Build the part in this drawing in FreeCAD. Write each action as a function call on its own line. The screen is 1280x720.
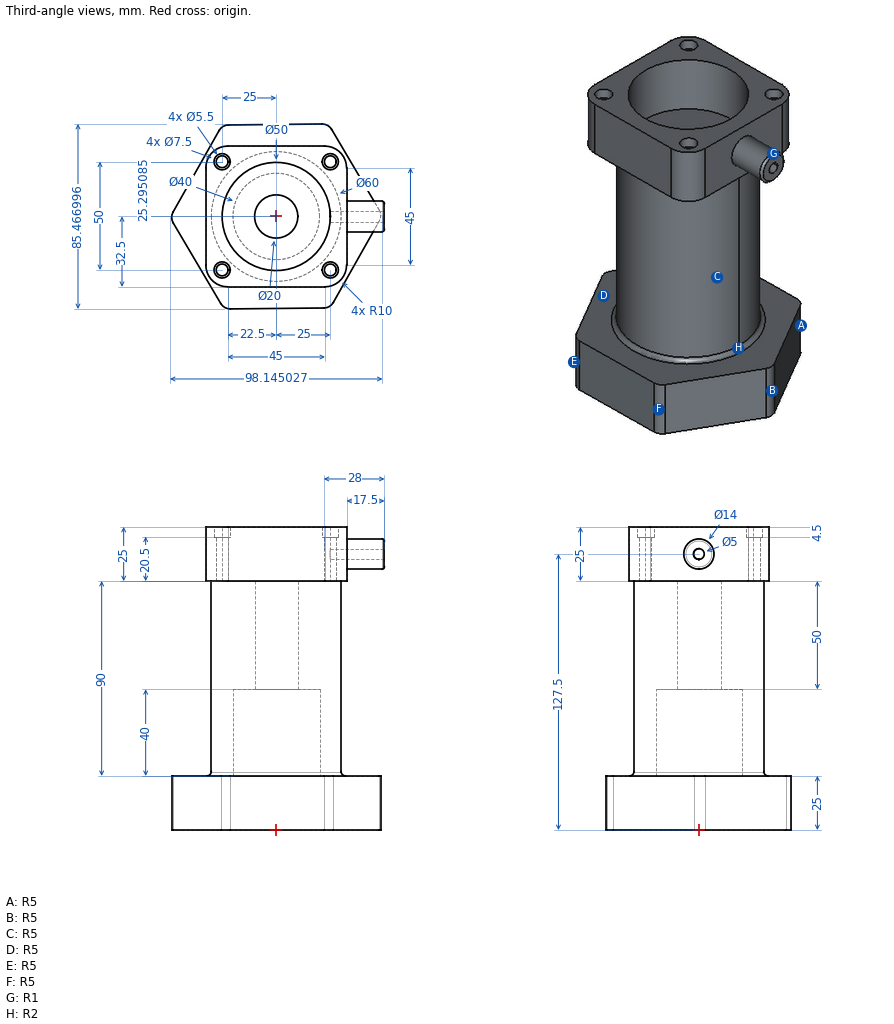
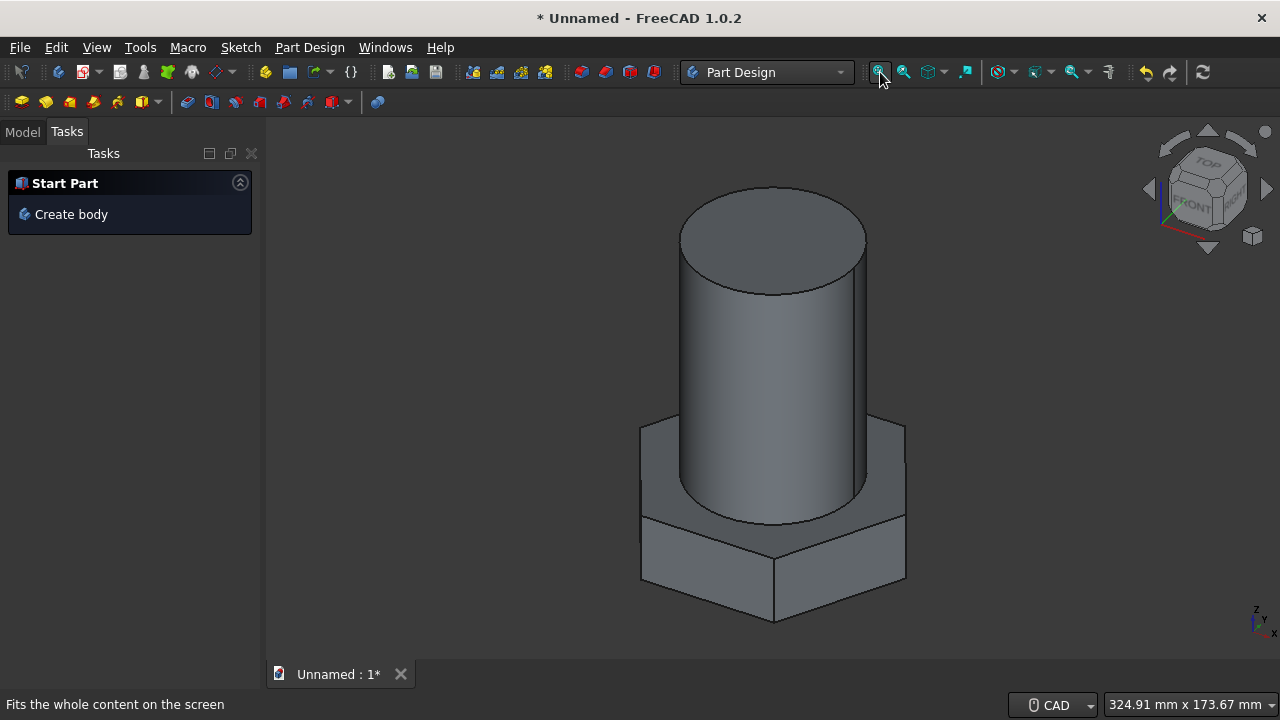
click(773, 240)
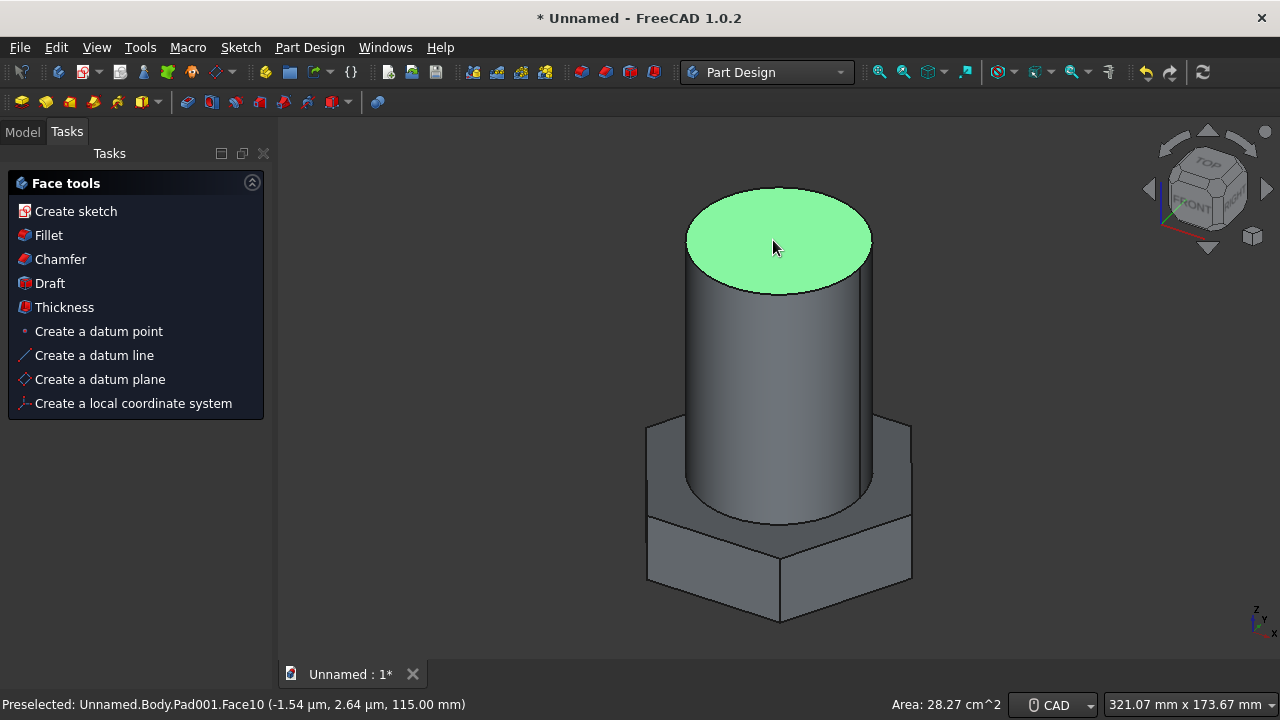
click(84, 72)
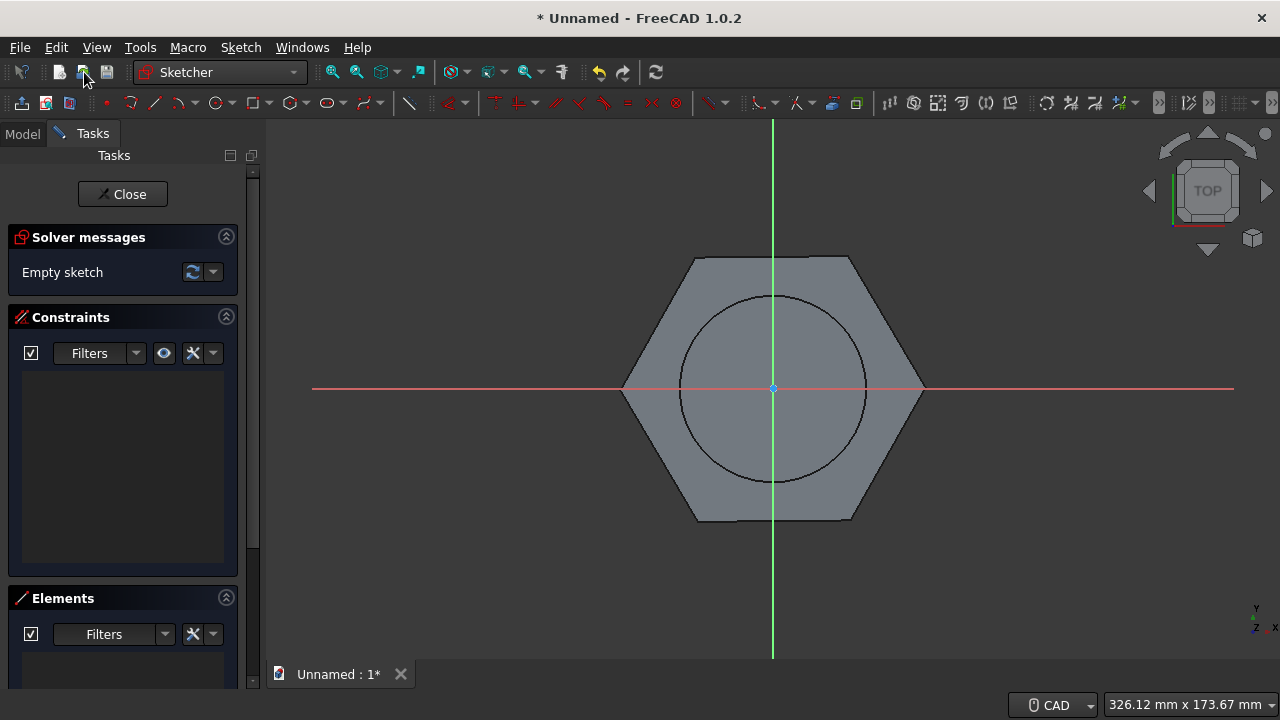
scroll(856, 389, up, 3)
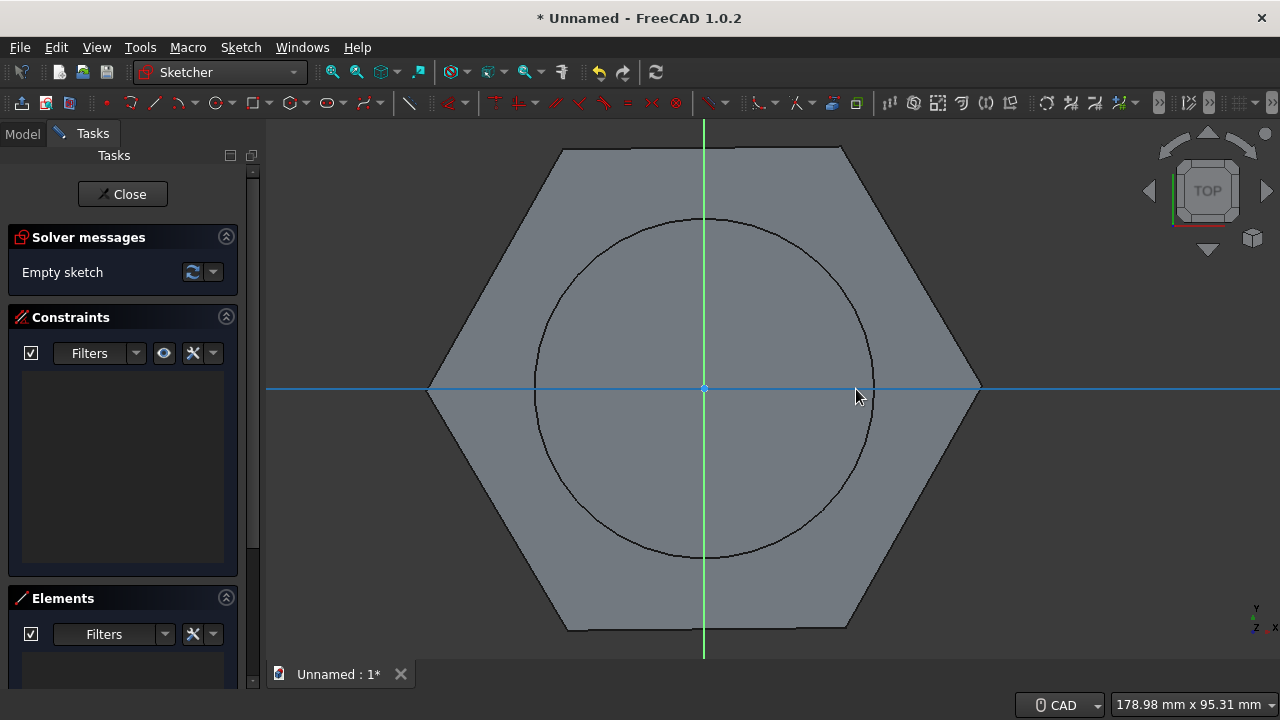
click(156, 104)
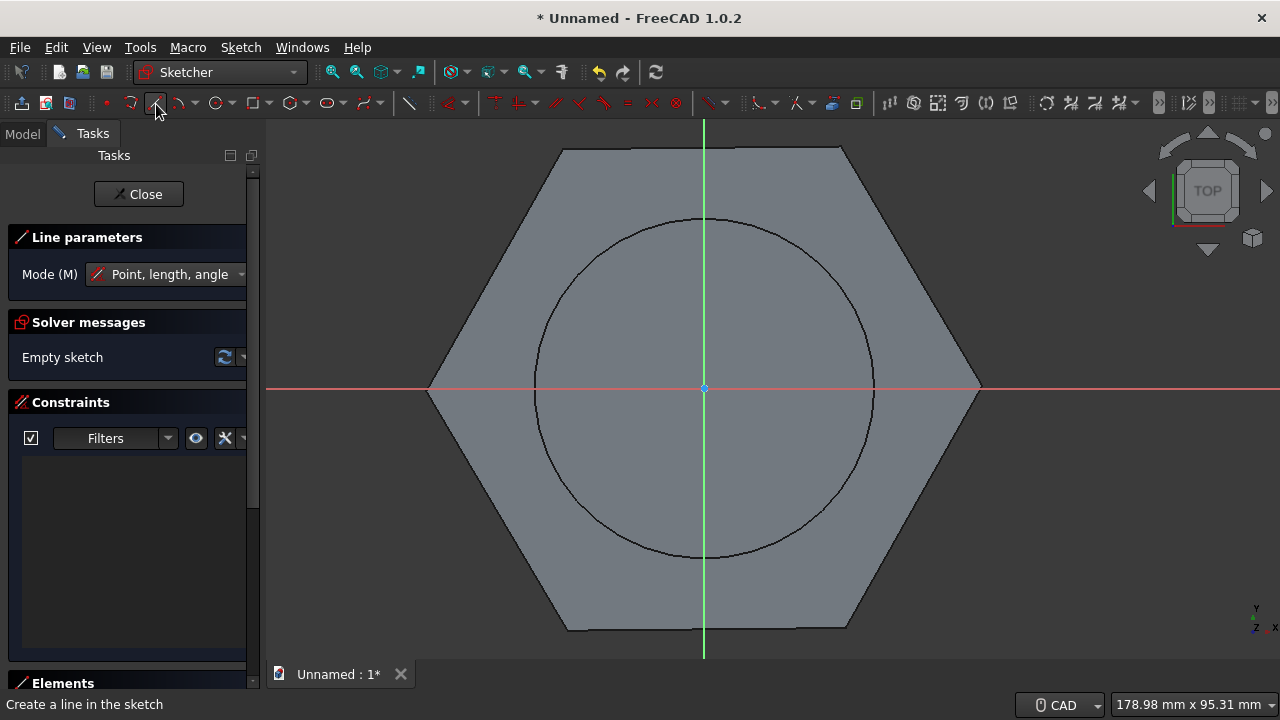
click(577, 573)
click(832, 573)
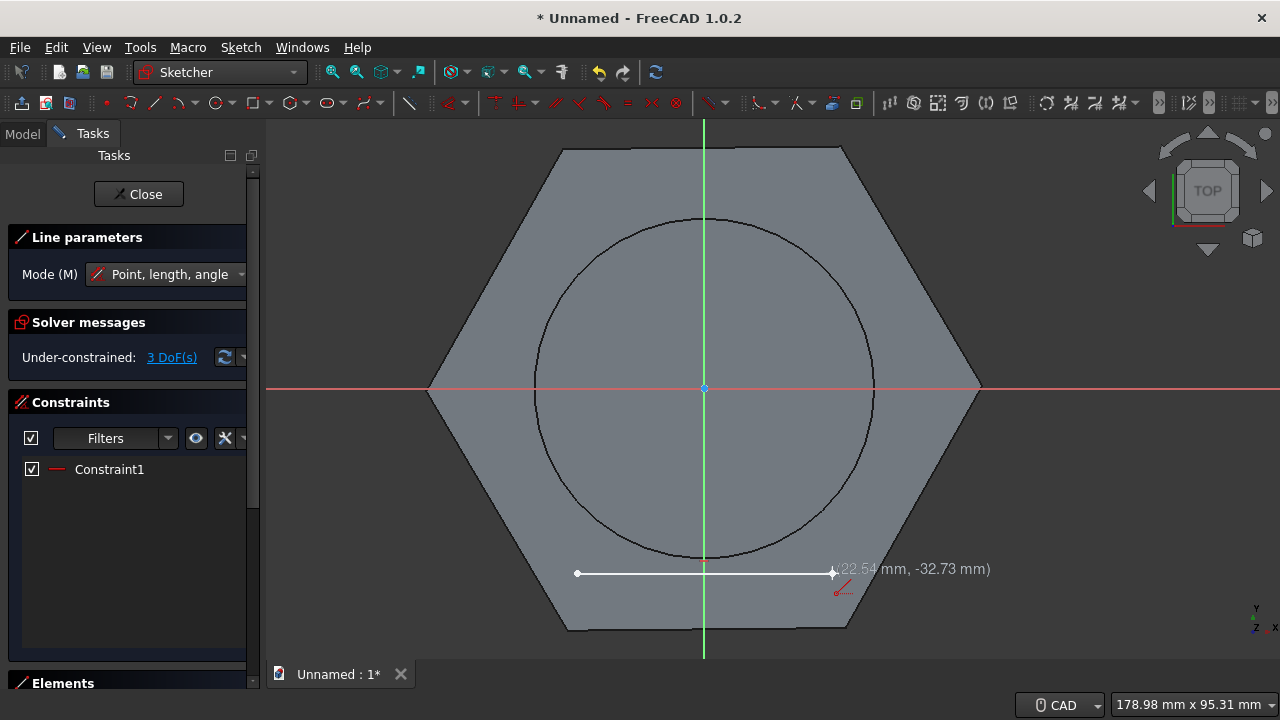
click(888, 516)
click(888, 261)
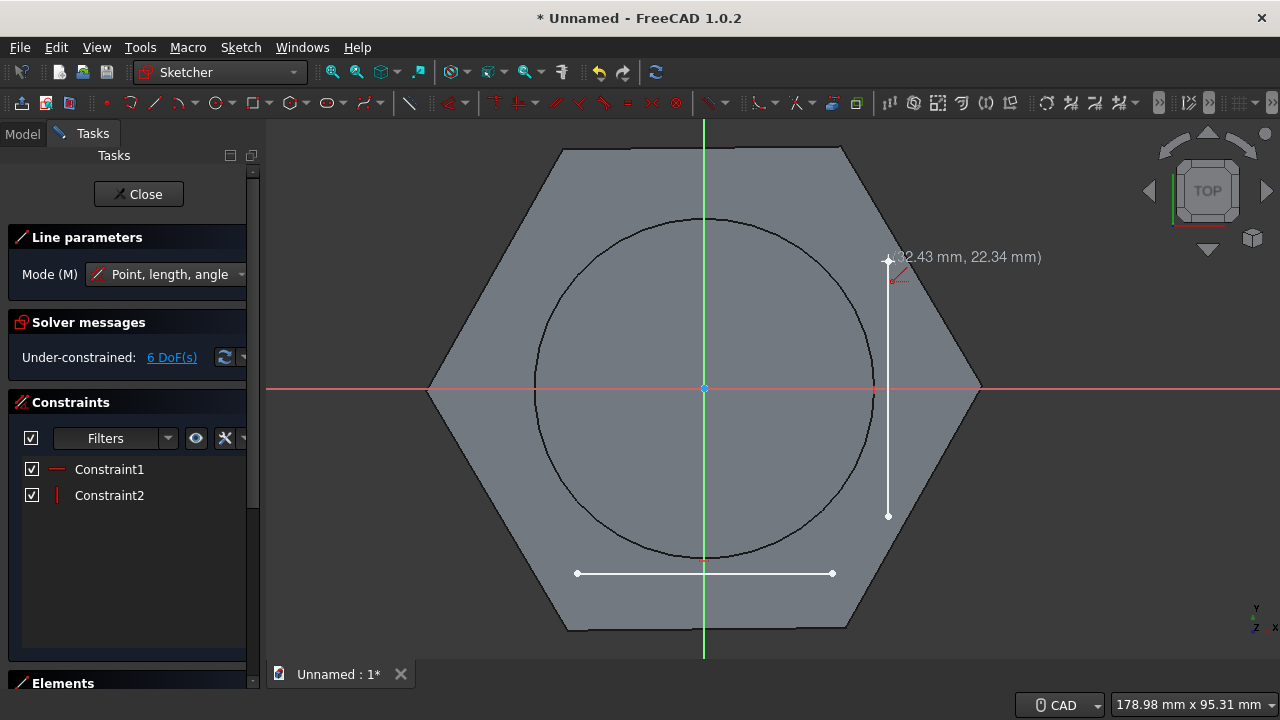
click(832, 204)
click(577, 204)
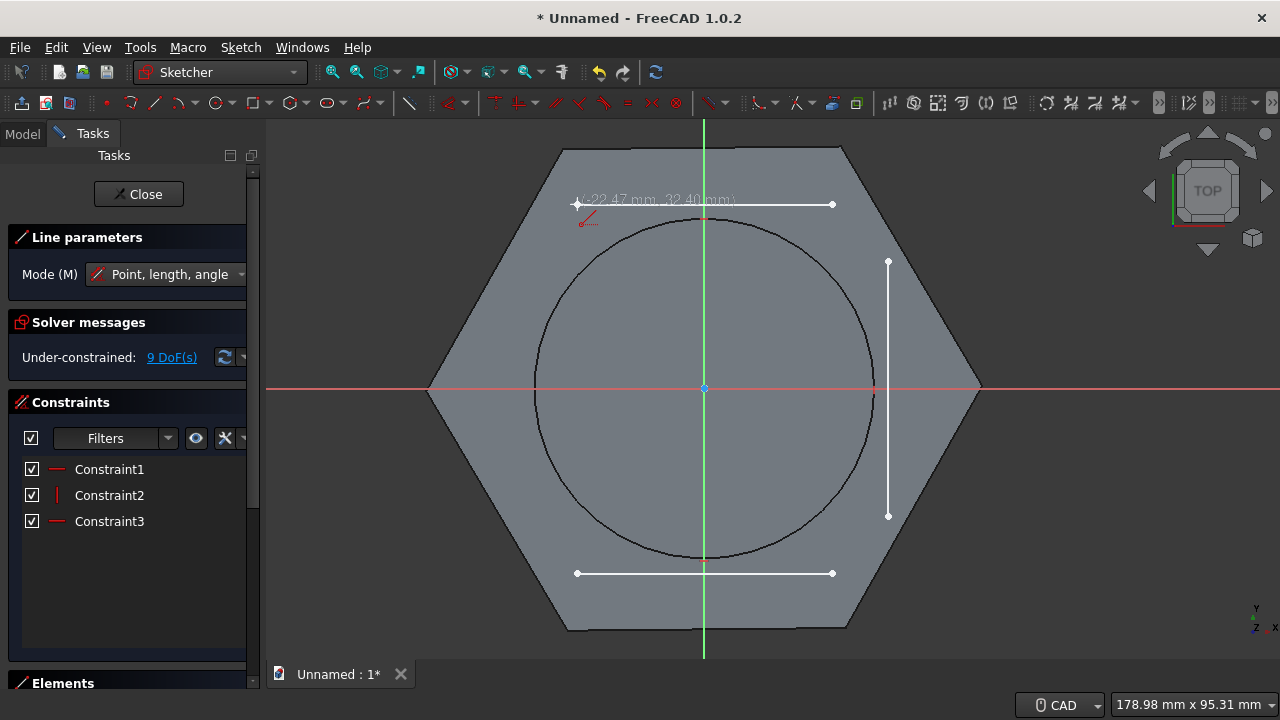
click(520, 261)
click(520, 516)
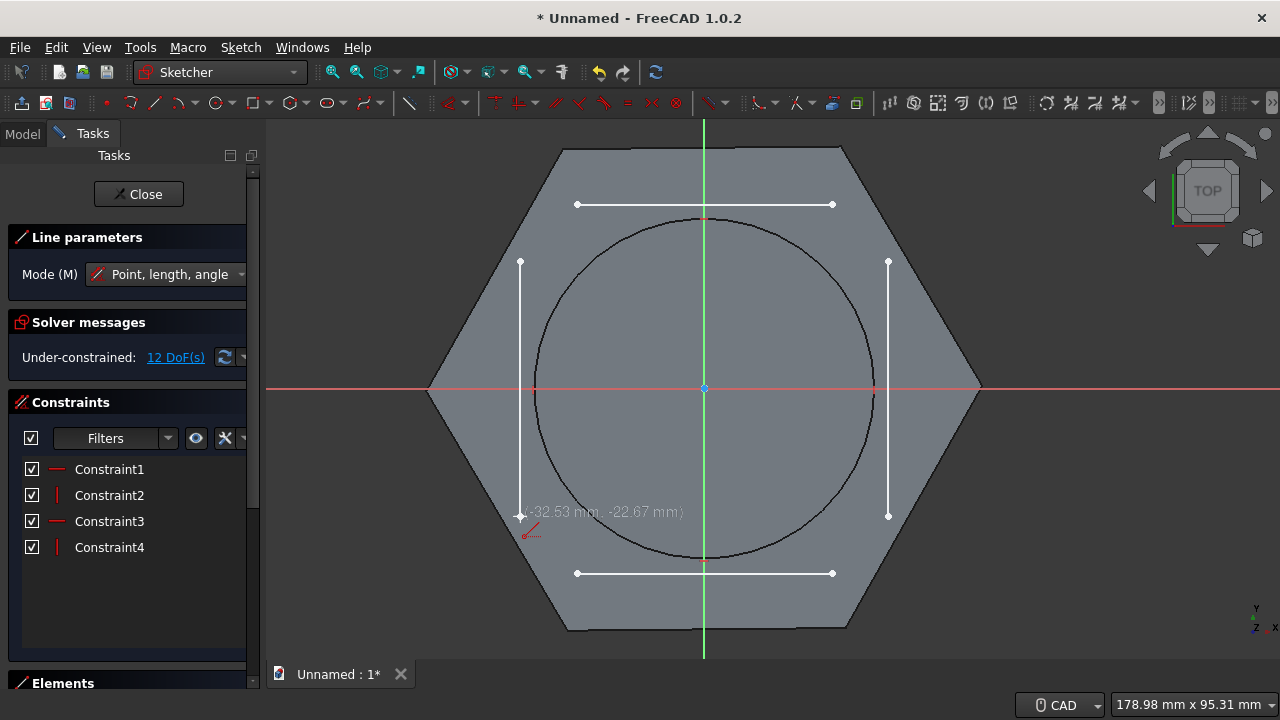
key(g)
key(3)
key(a)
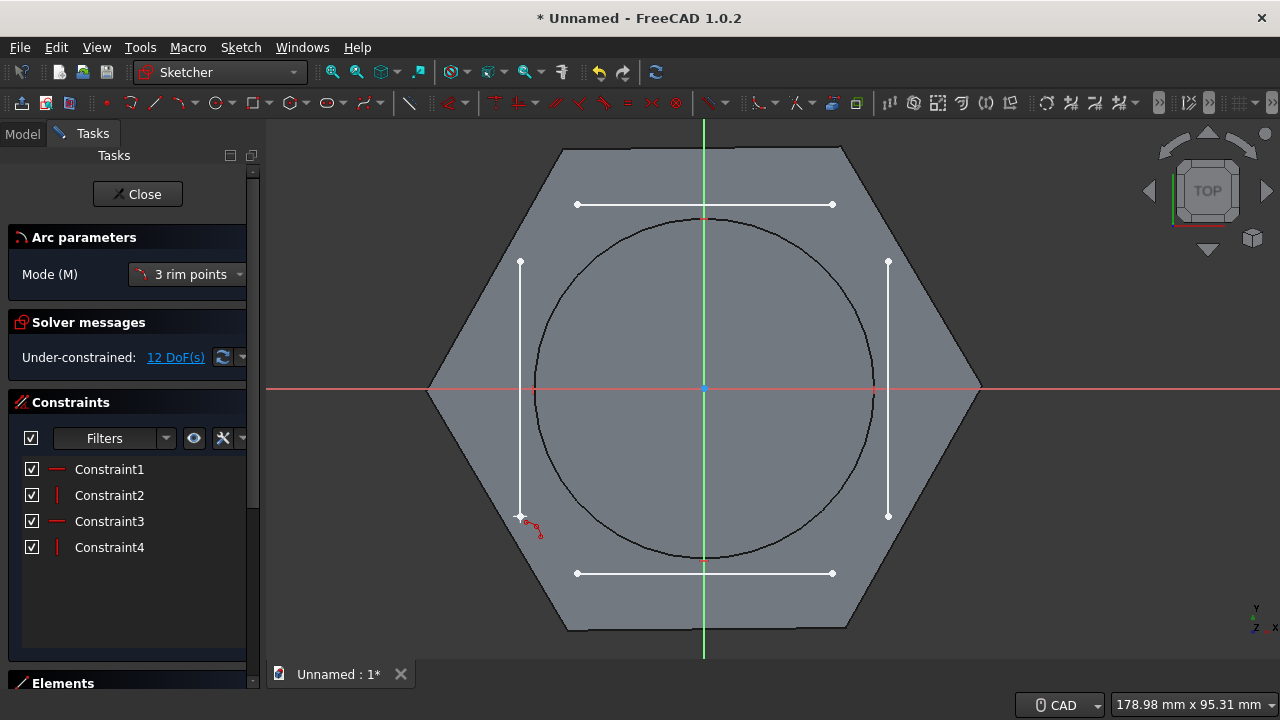
click(832, 574)
click(888, 517)
click(872, 556)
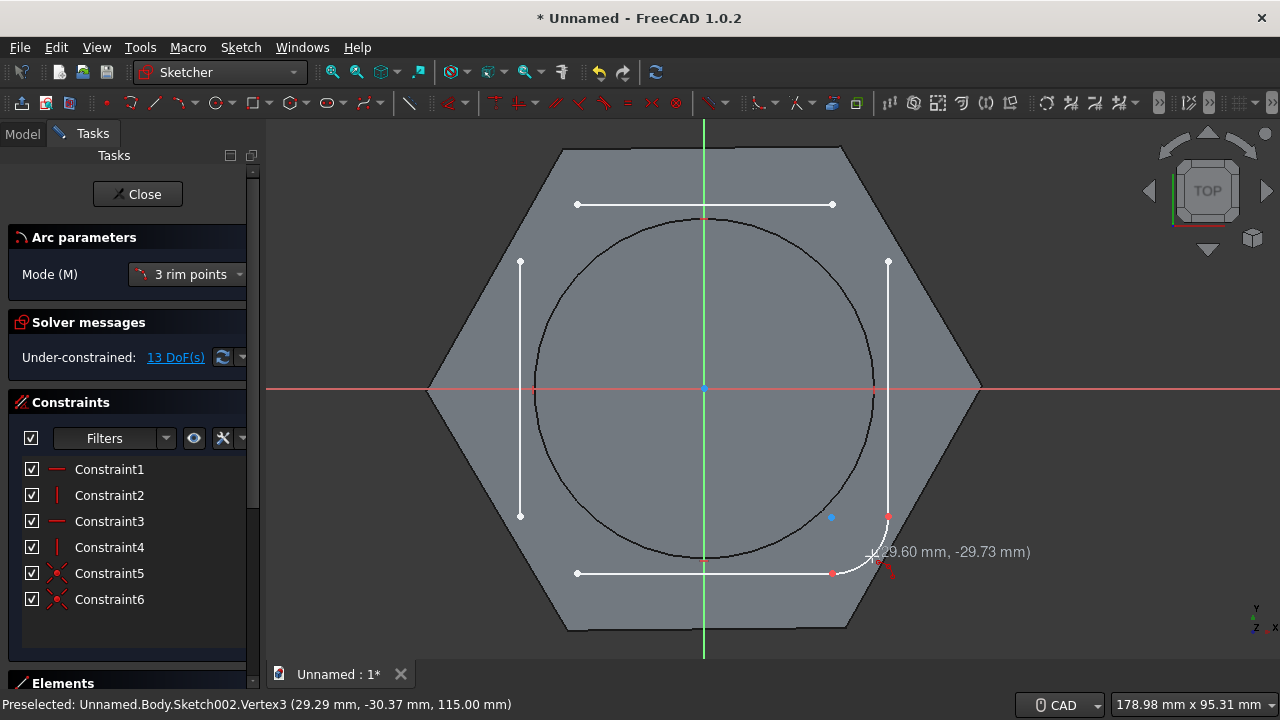
click(888, 262)
click(832, 205)
click(872, 221)